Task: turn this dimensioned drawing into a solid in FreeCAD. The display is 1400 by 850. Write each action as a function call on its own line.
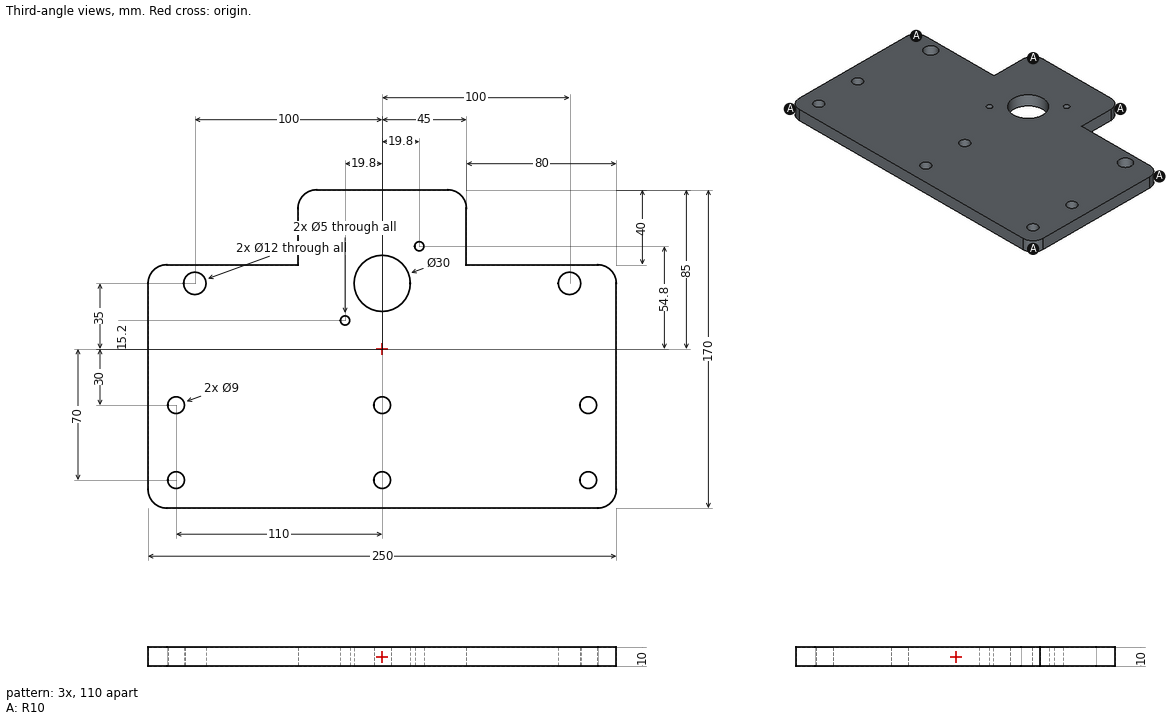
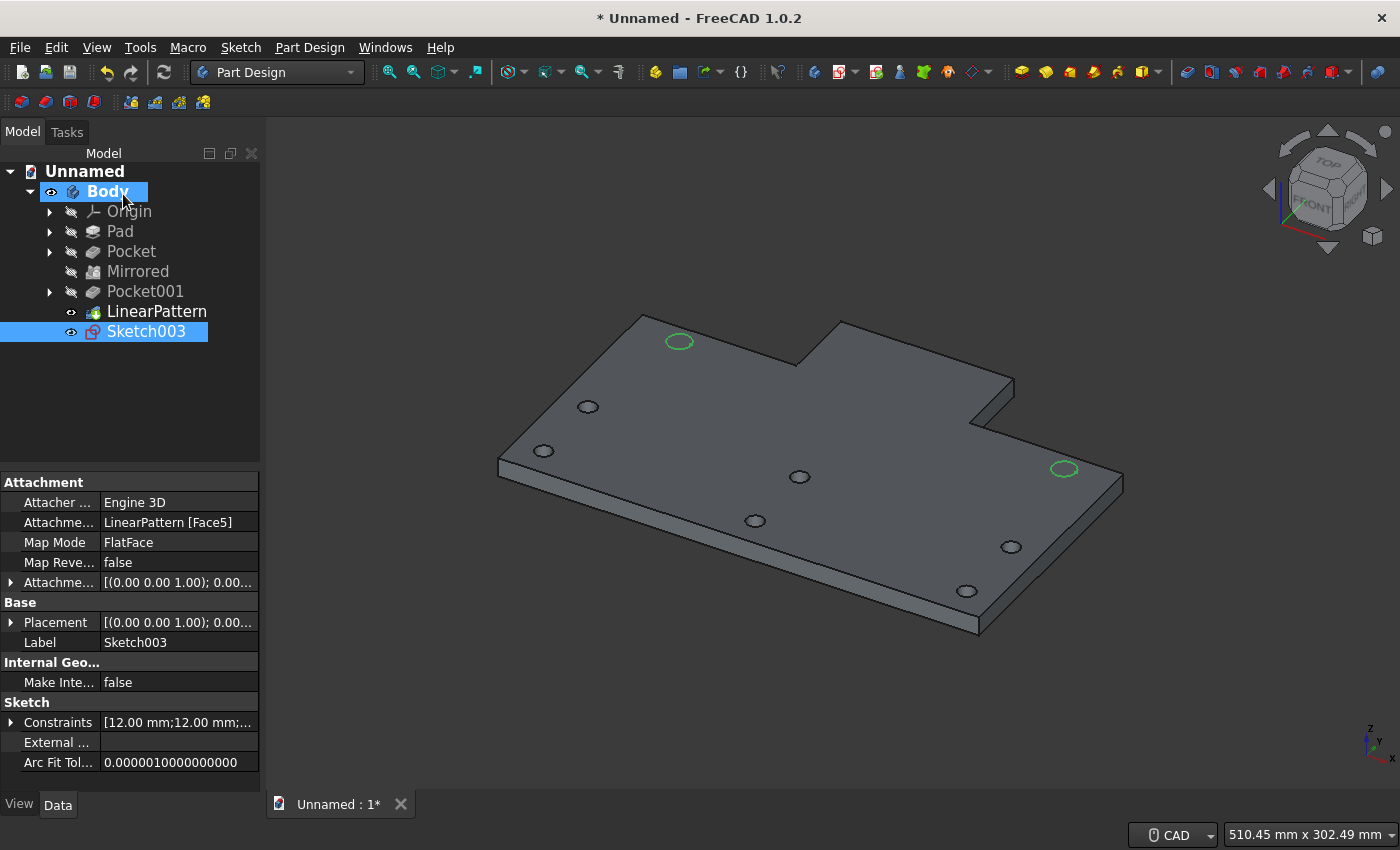
click(1212, 72)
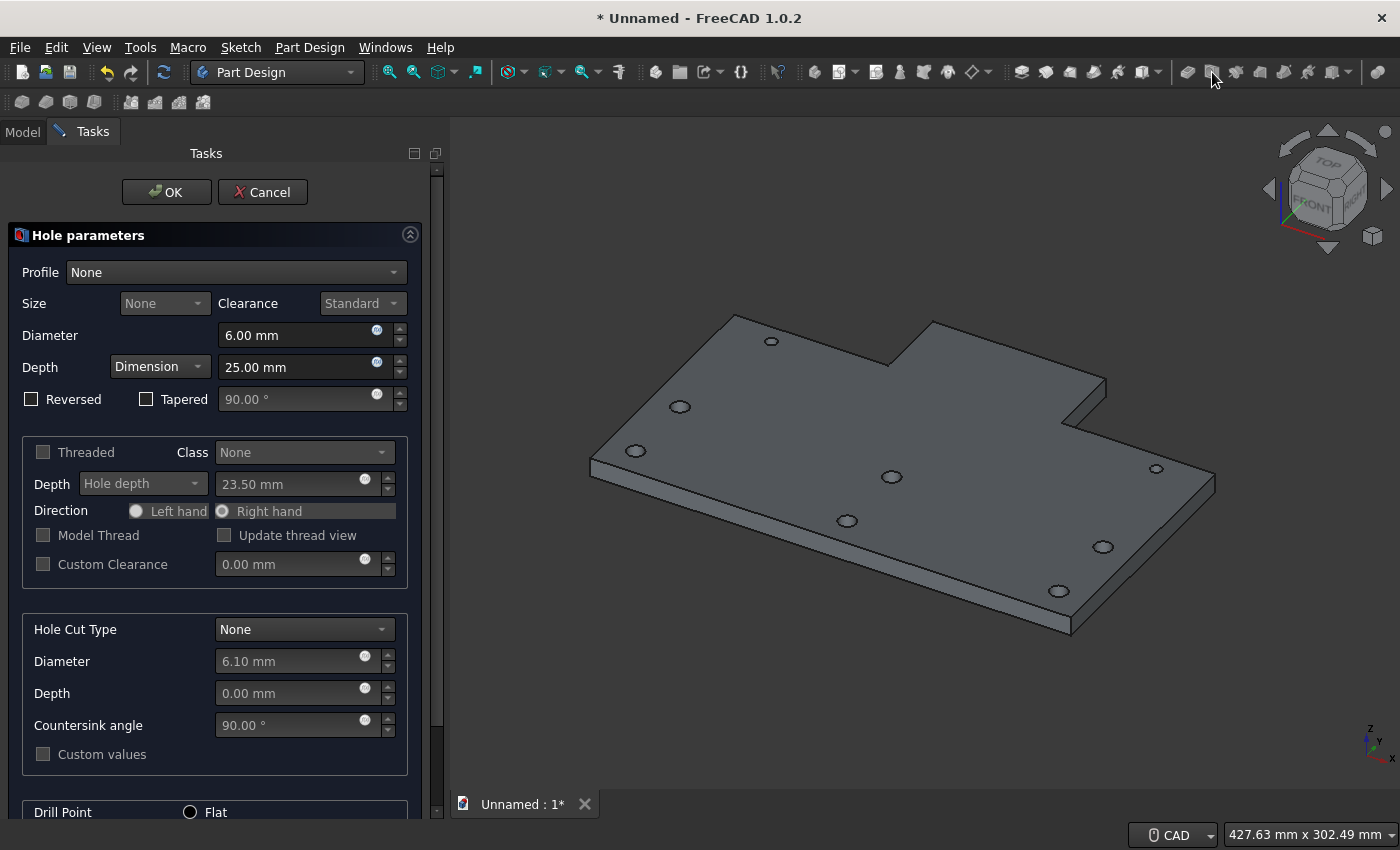
triple_click(305, 335)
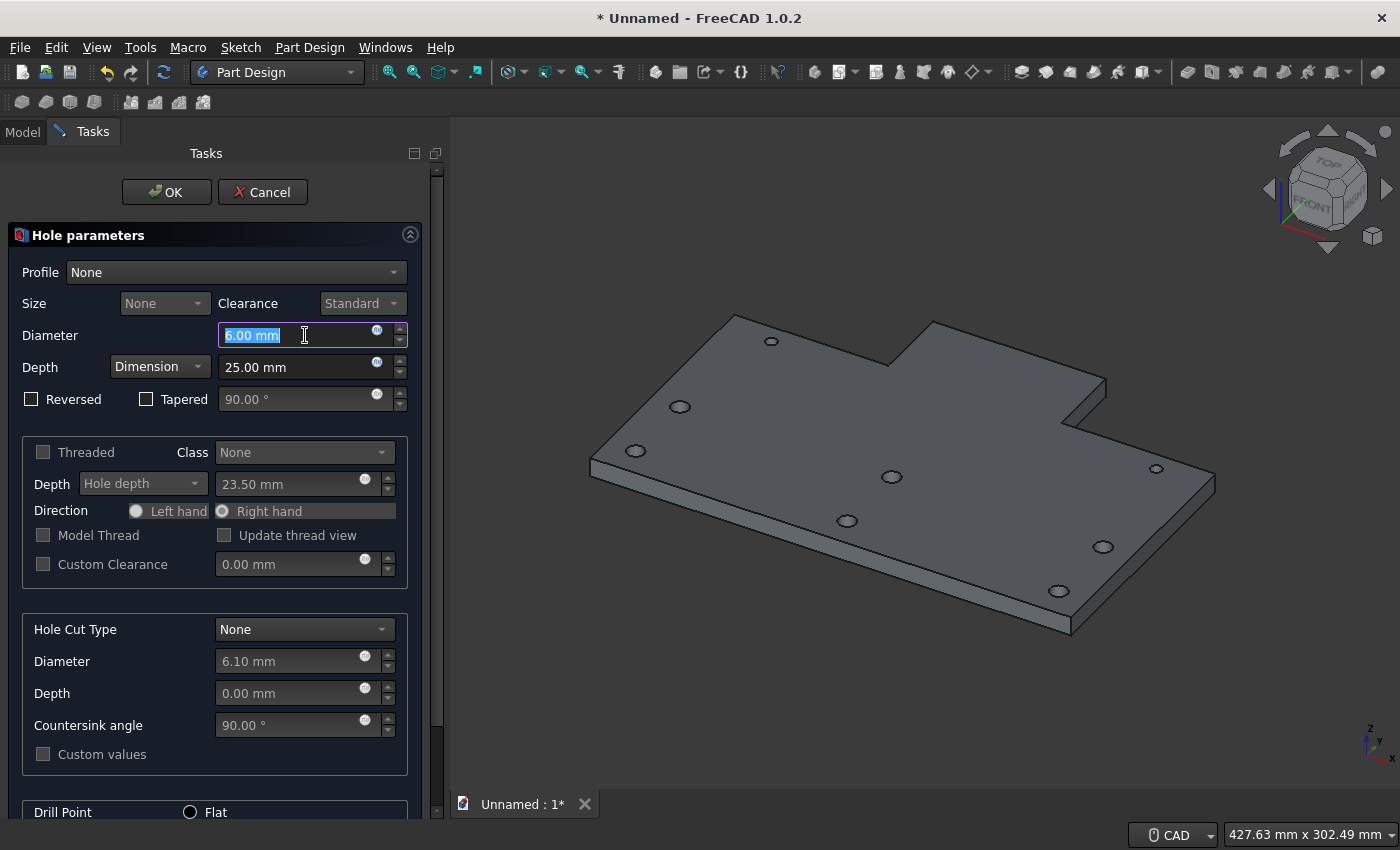
text(12)
key(Tab)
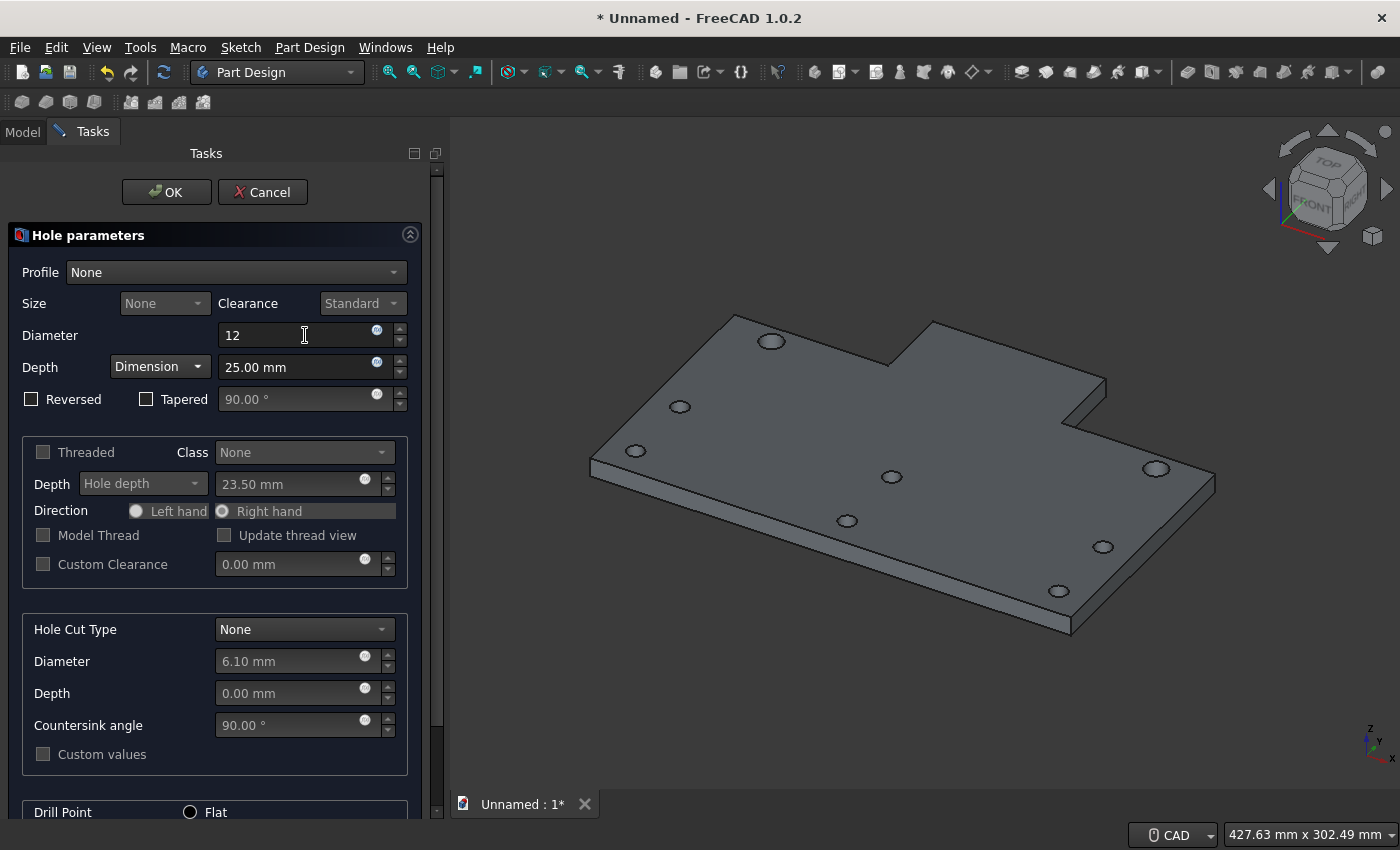
click(161, 366)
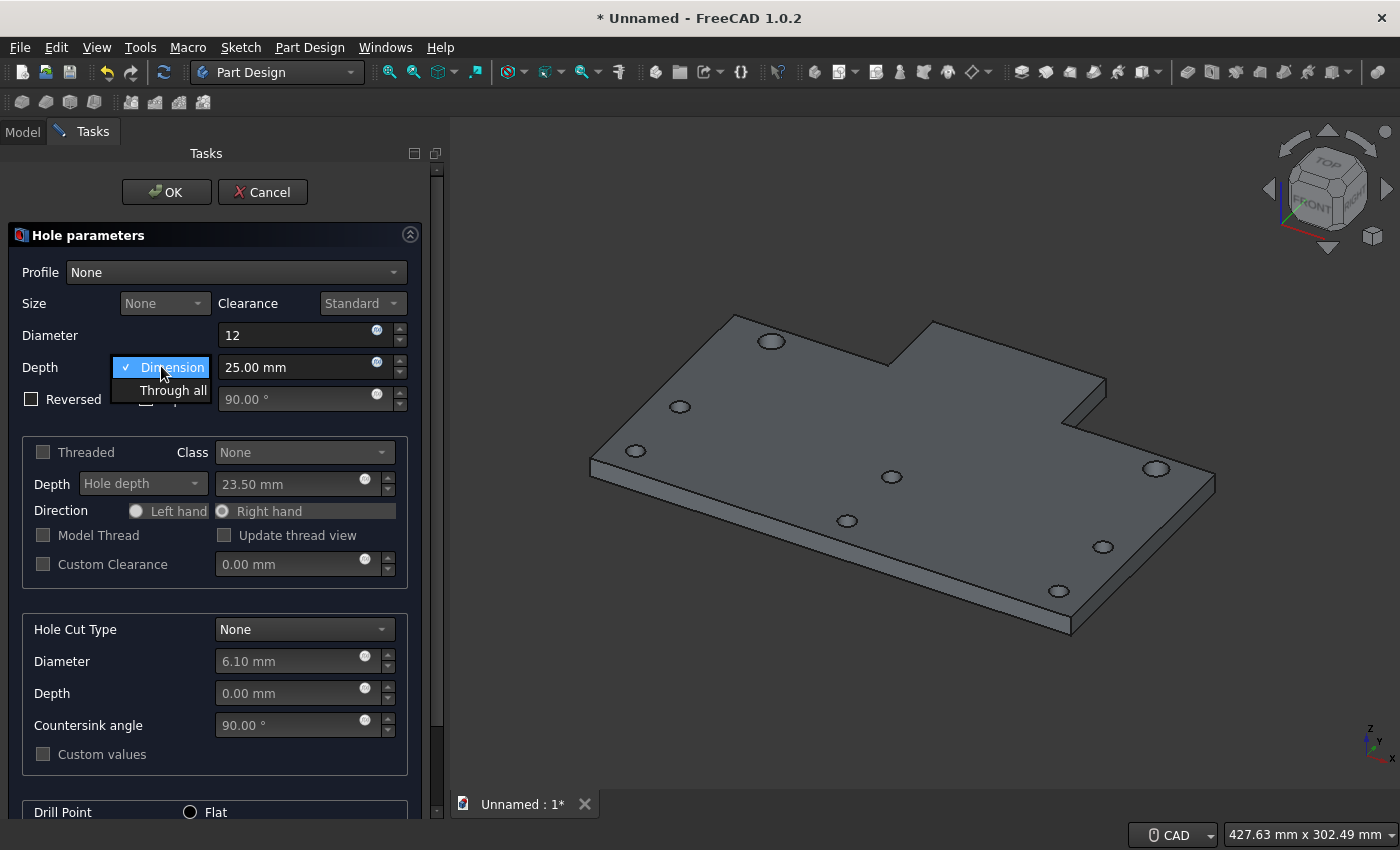
click(160, 390)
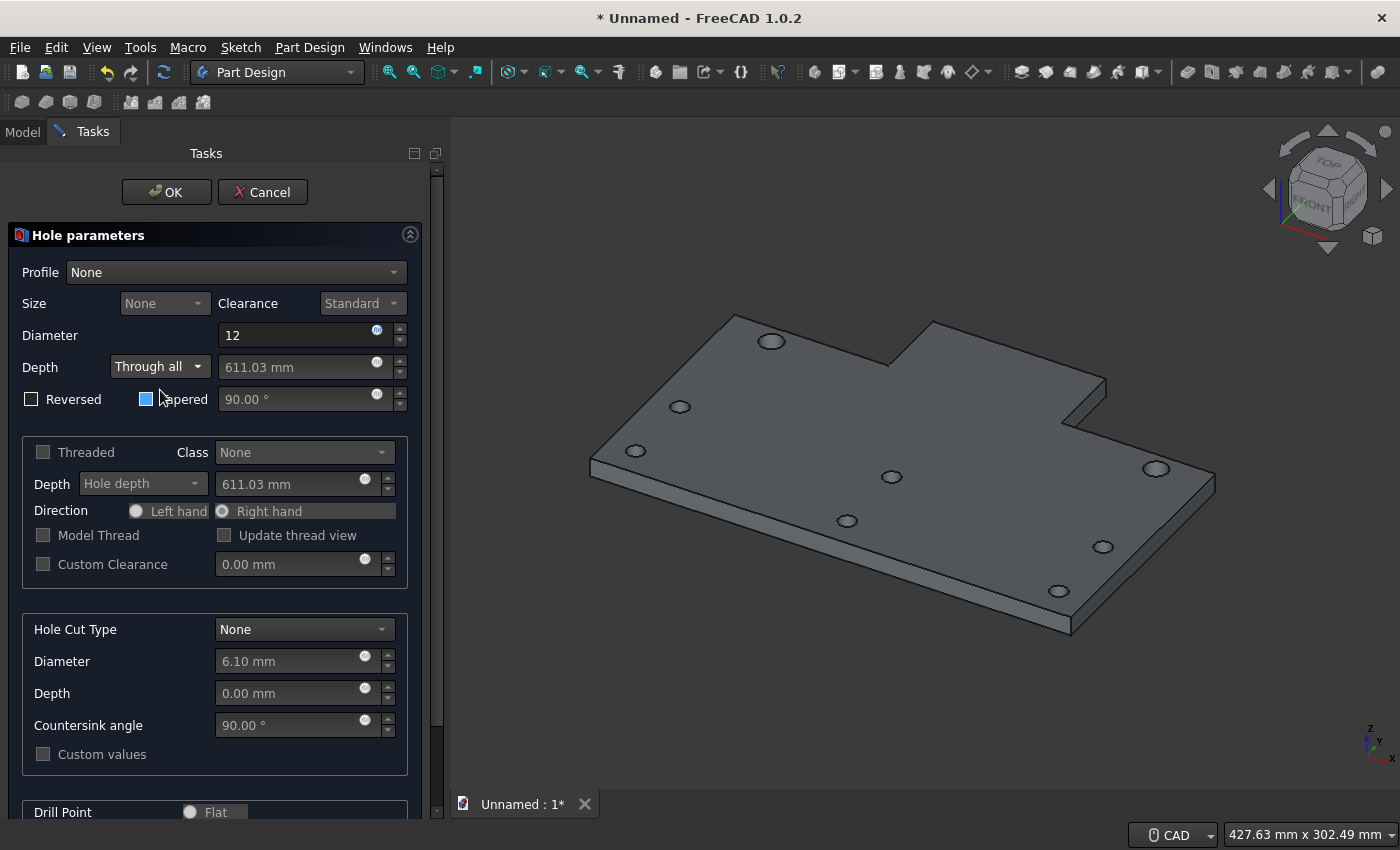
click(167, 192)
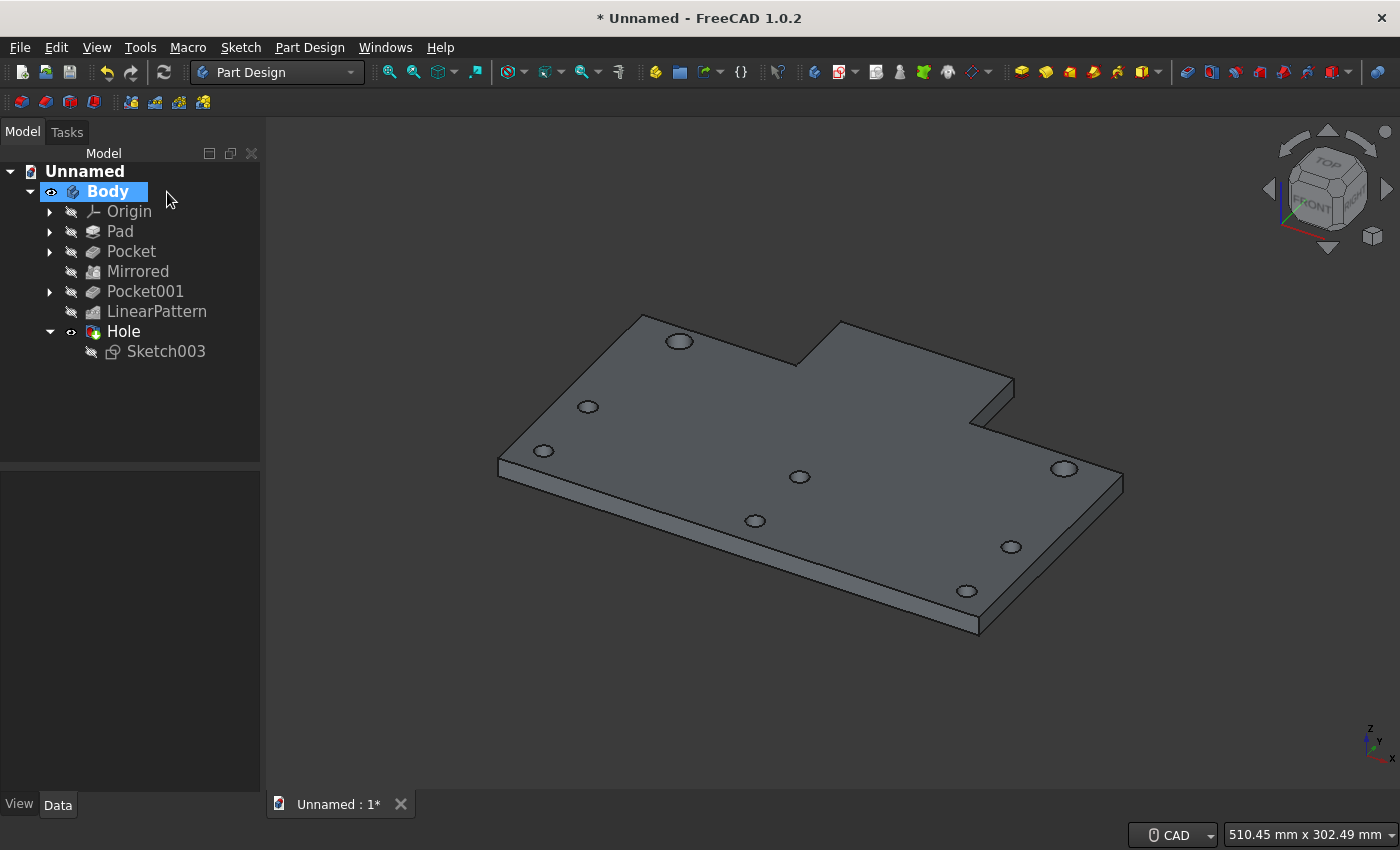
click(860, 416)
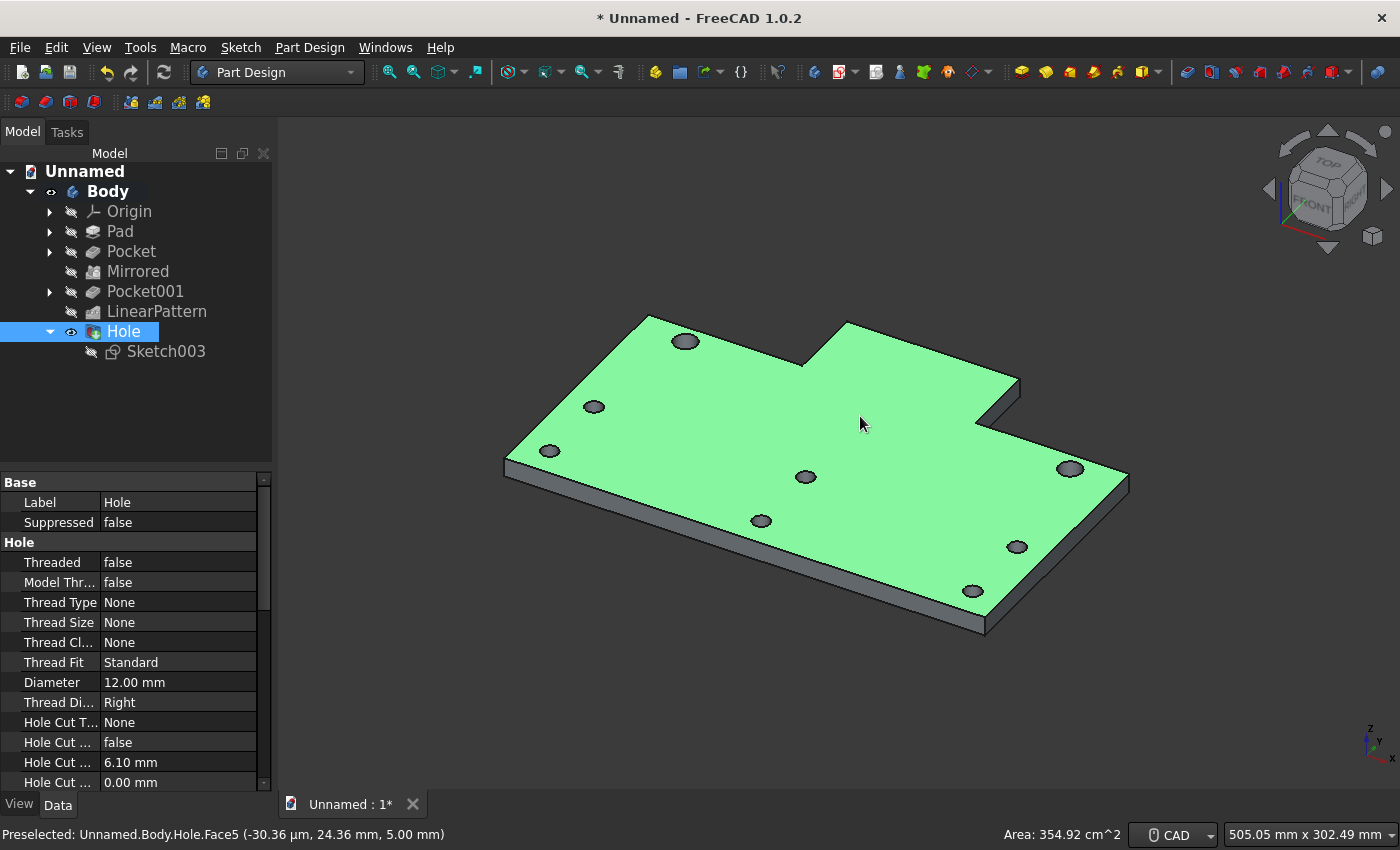
click(840, 72)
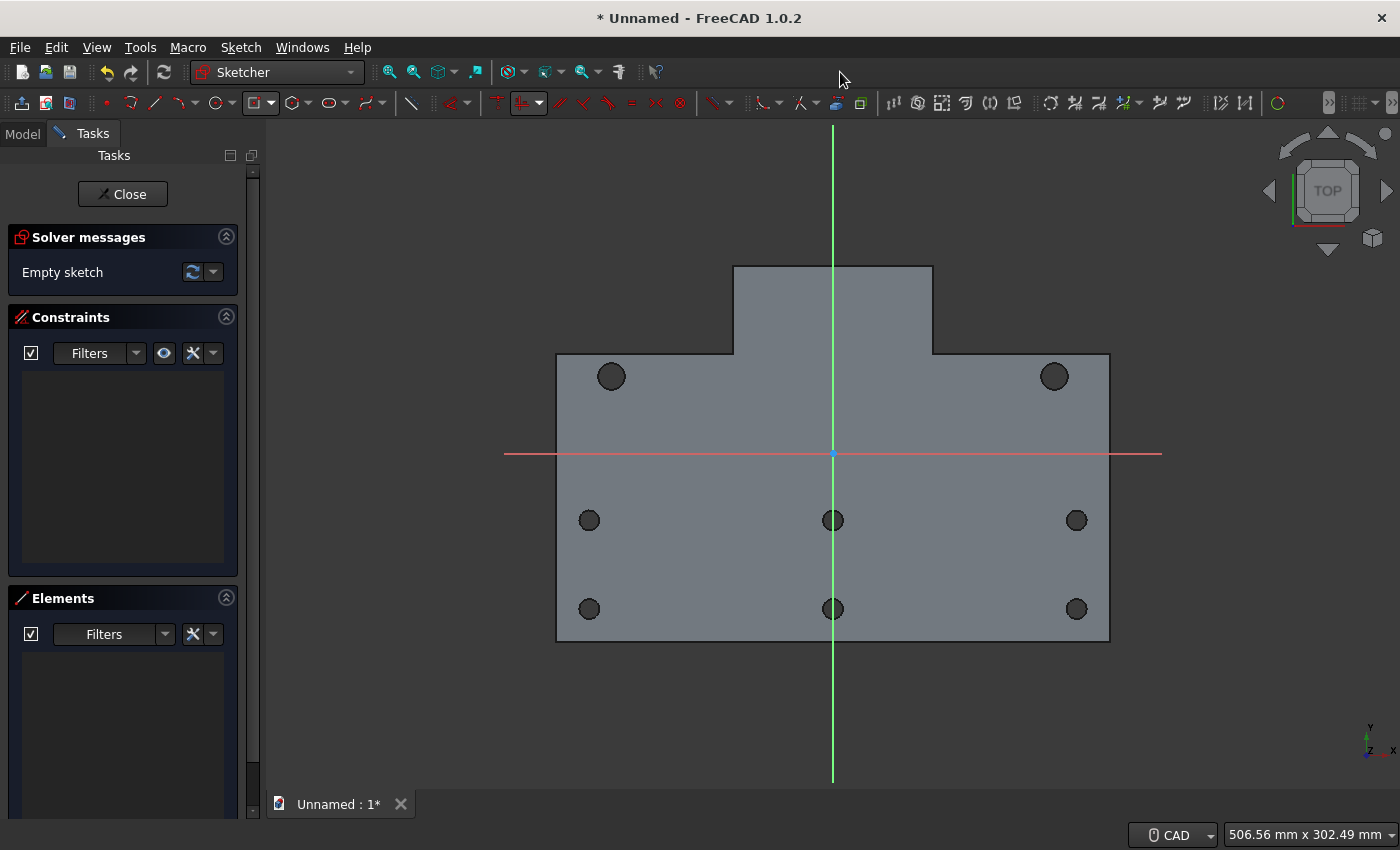
scroll(855, 381, up, 7)